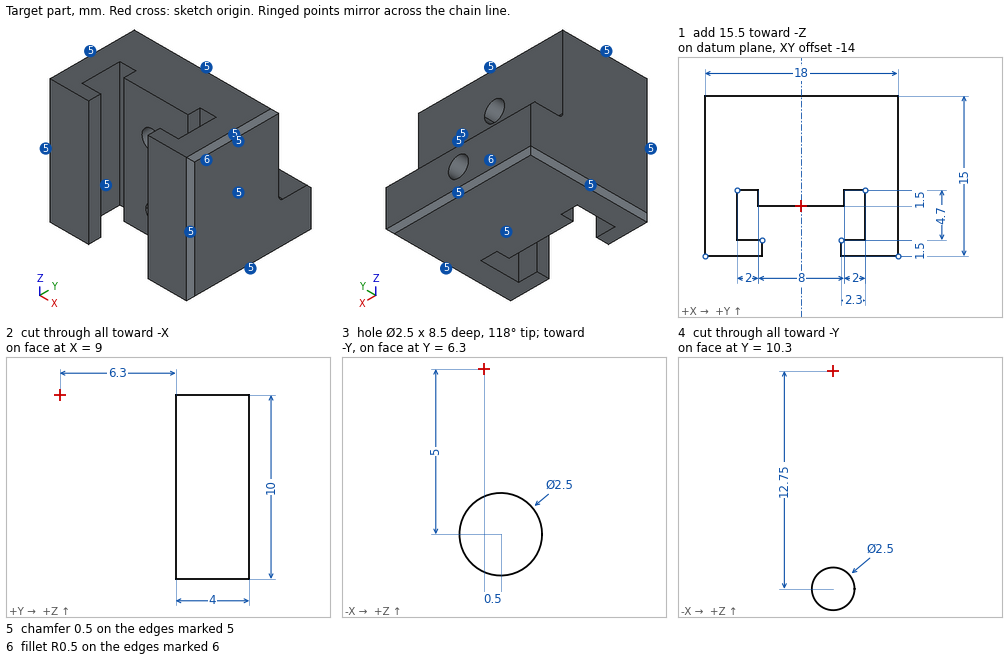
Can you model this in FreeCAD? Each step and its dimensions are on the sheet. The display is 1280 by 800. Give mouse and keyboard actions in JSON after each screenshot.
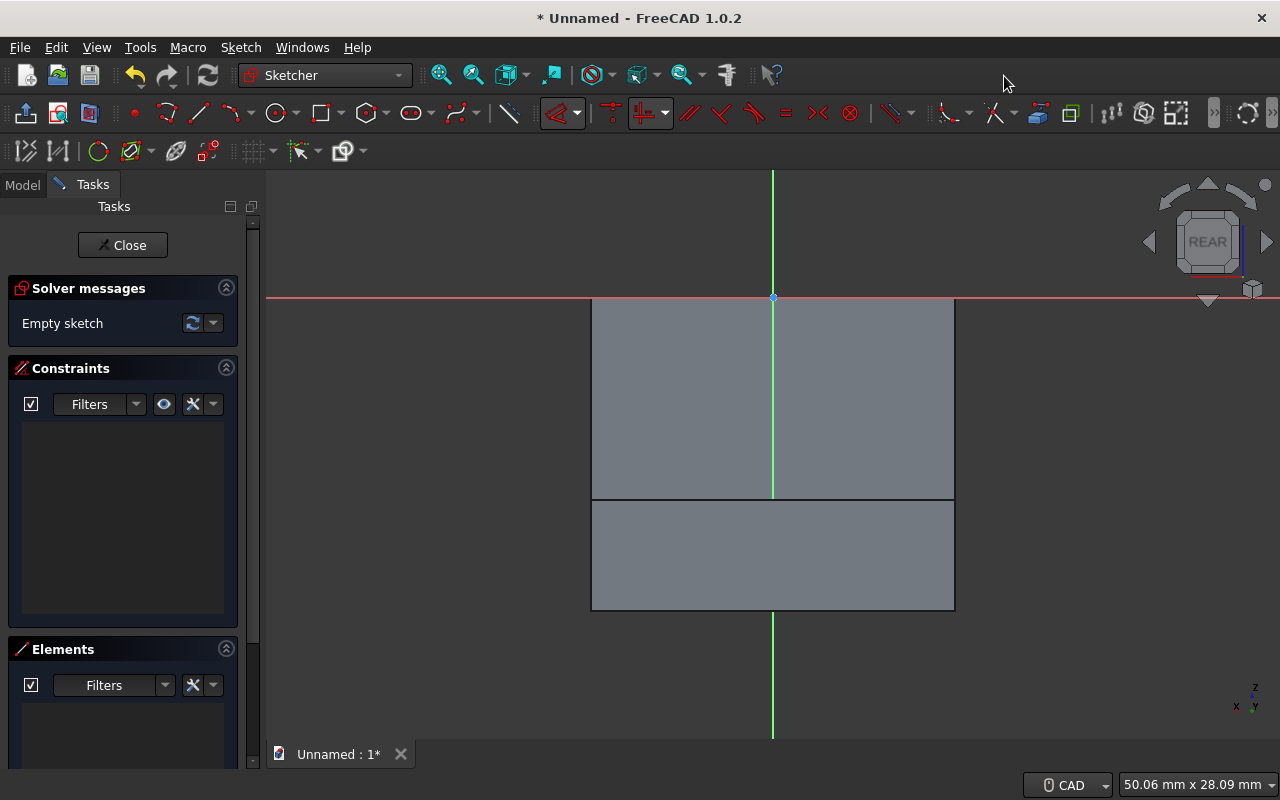
{"action": "scroll", "coordinate": [795, 390], "scroll_direction": "up", "scroll_amount": 10}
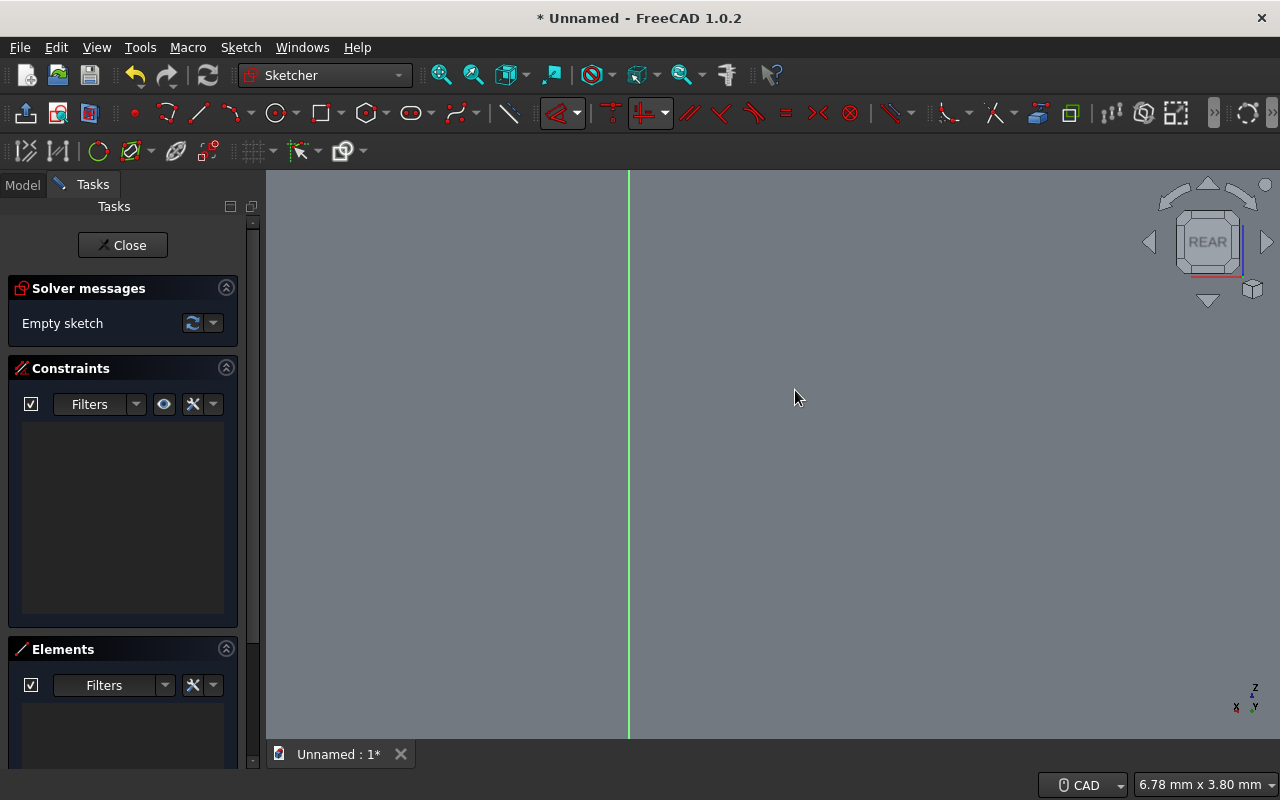
{"action": "key", "text": "g c"}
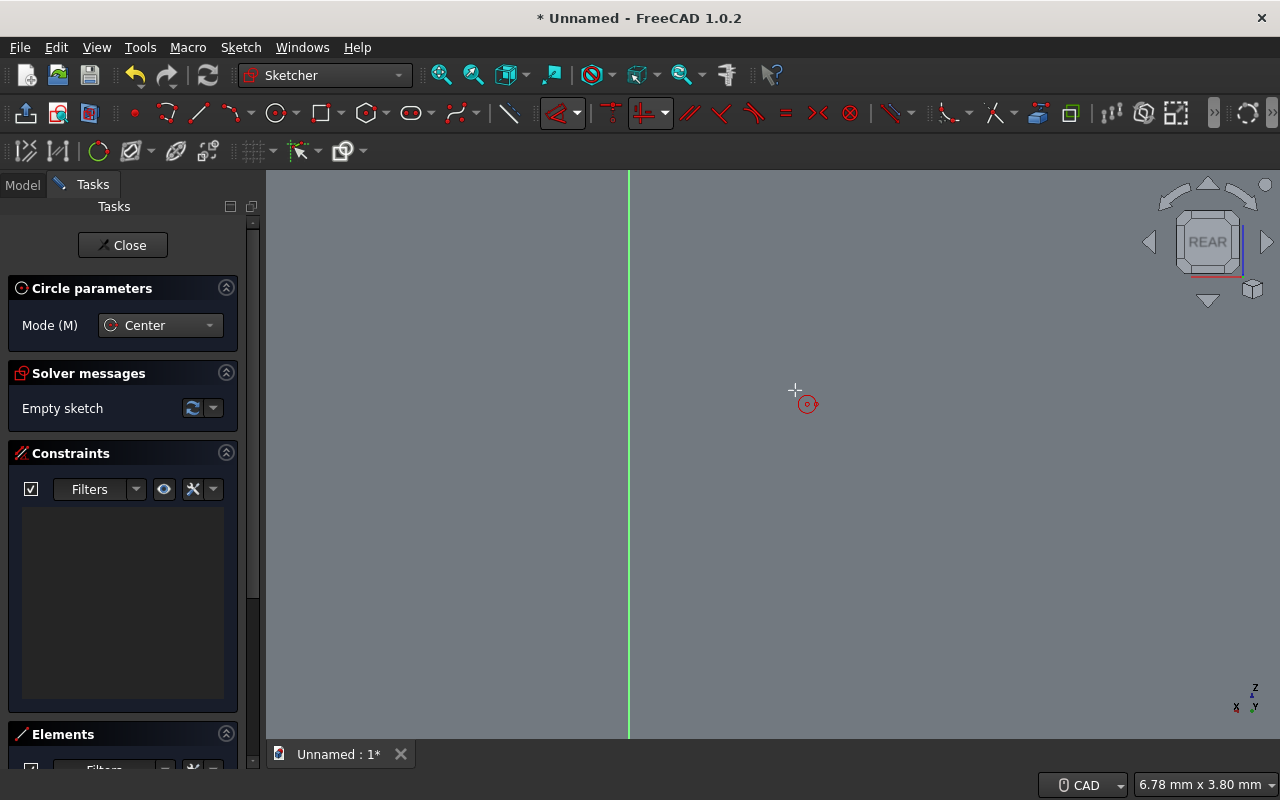
{"action": "left_click", "coordinate": [704, 453]}
{"action": "mouse_move", "coordinate": [836, 320]}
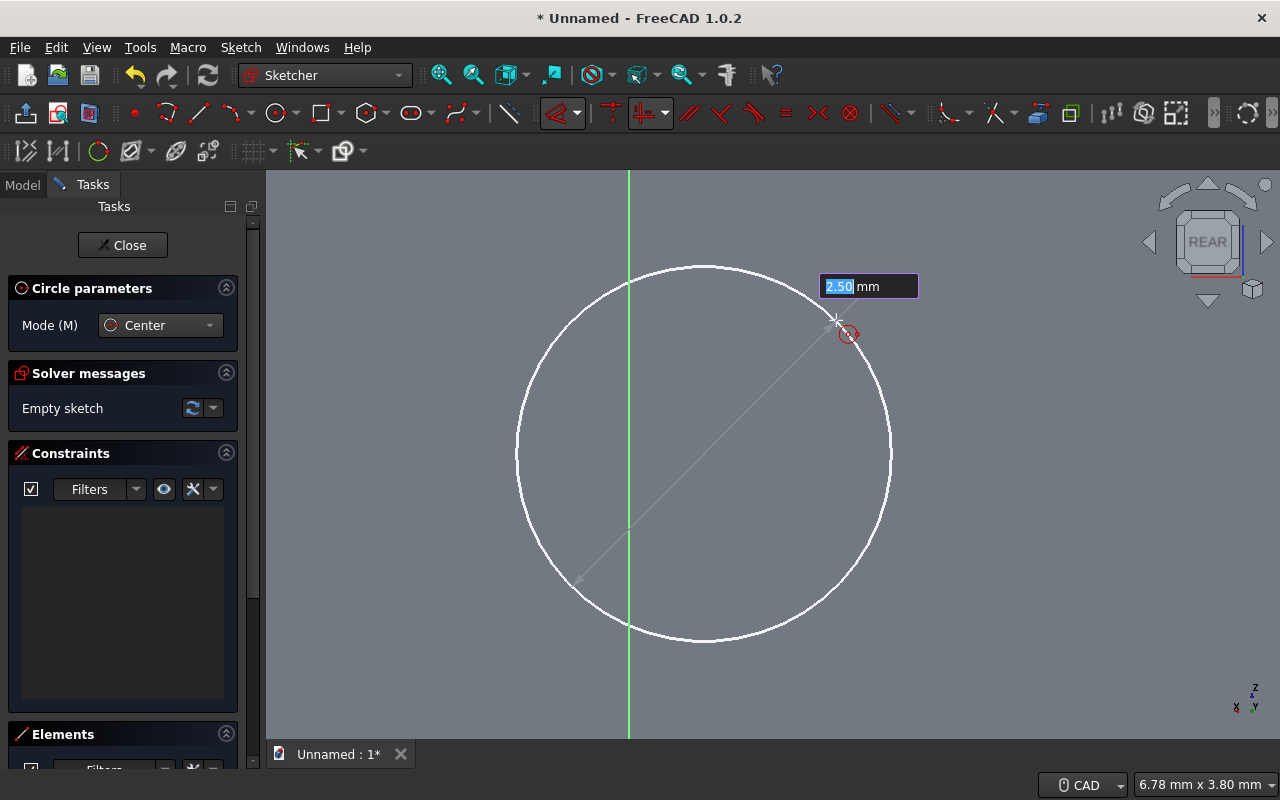
{"action": "type", "text": "2.5"}
{"action": "key", "text": "Return"}
{"action": "key", "text": "Escape"}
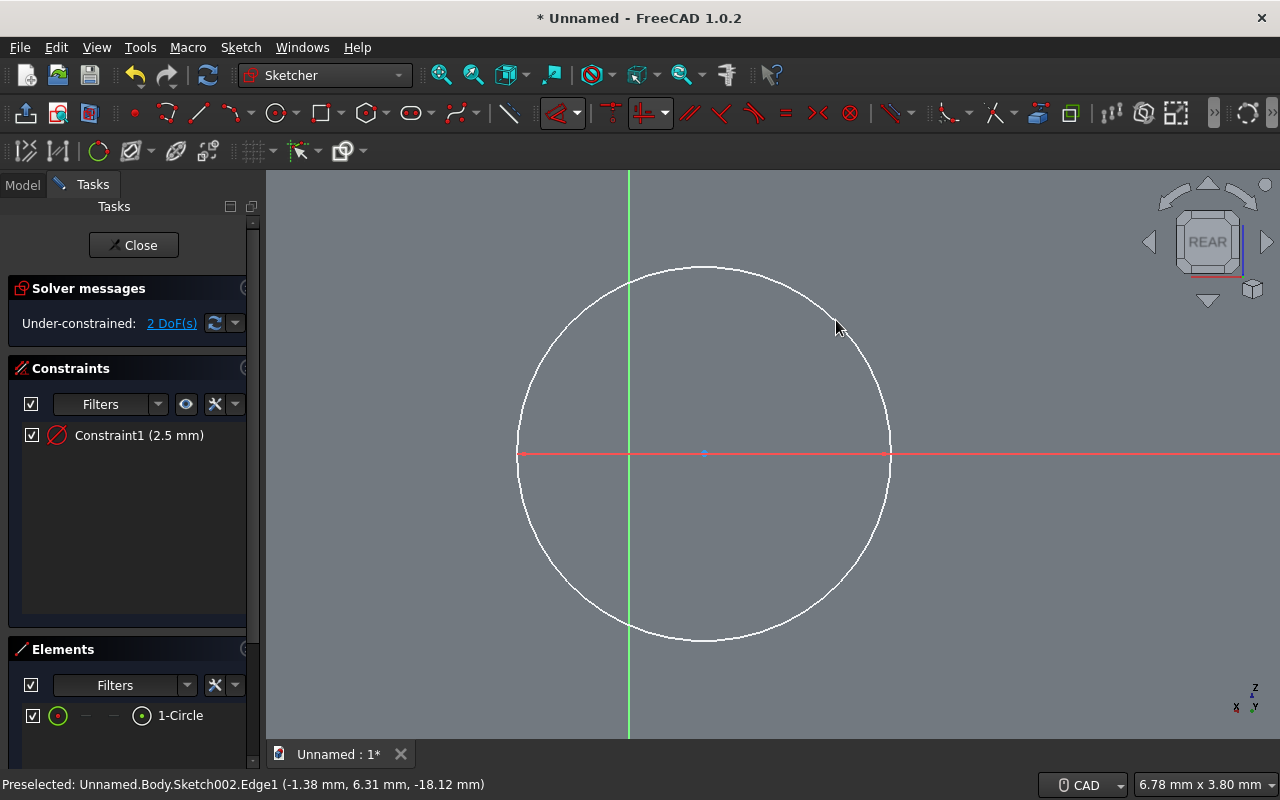
{"action": "left_click", "coordinate": [556, 114]}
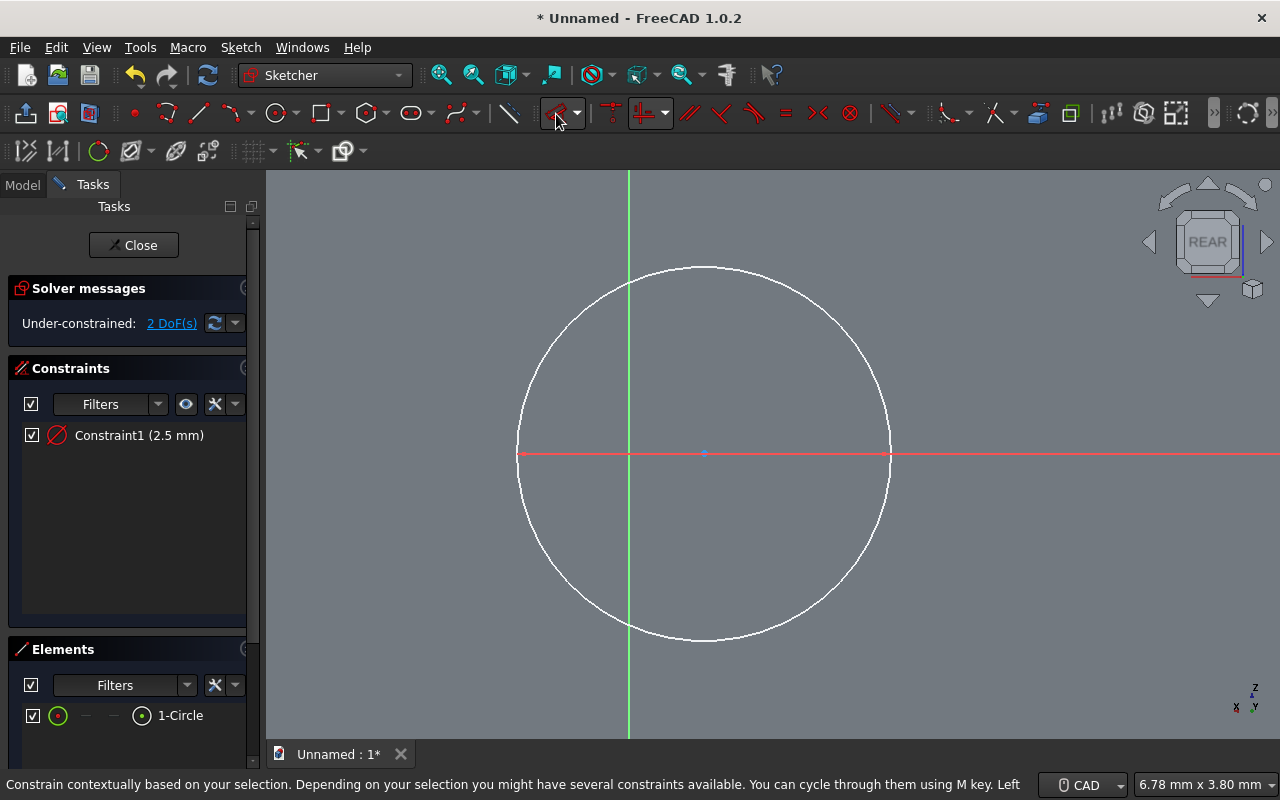
{"action": "left_click", "coordinate": [704, 454]}
{"action": "left_click", "coordinate": [595, 326]}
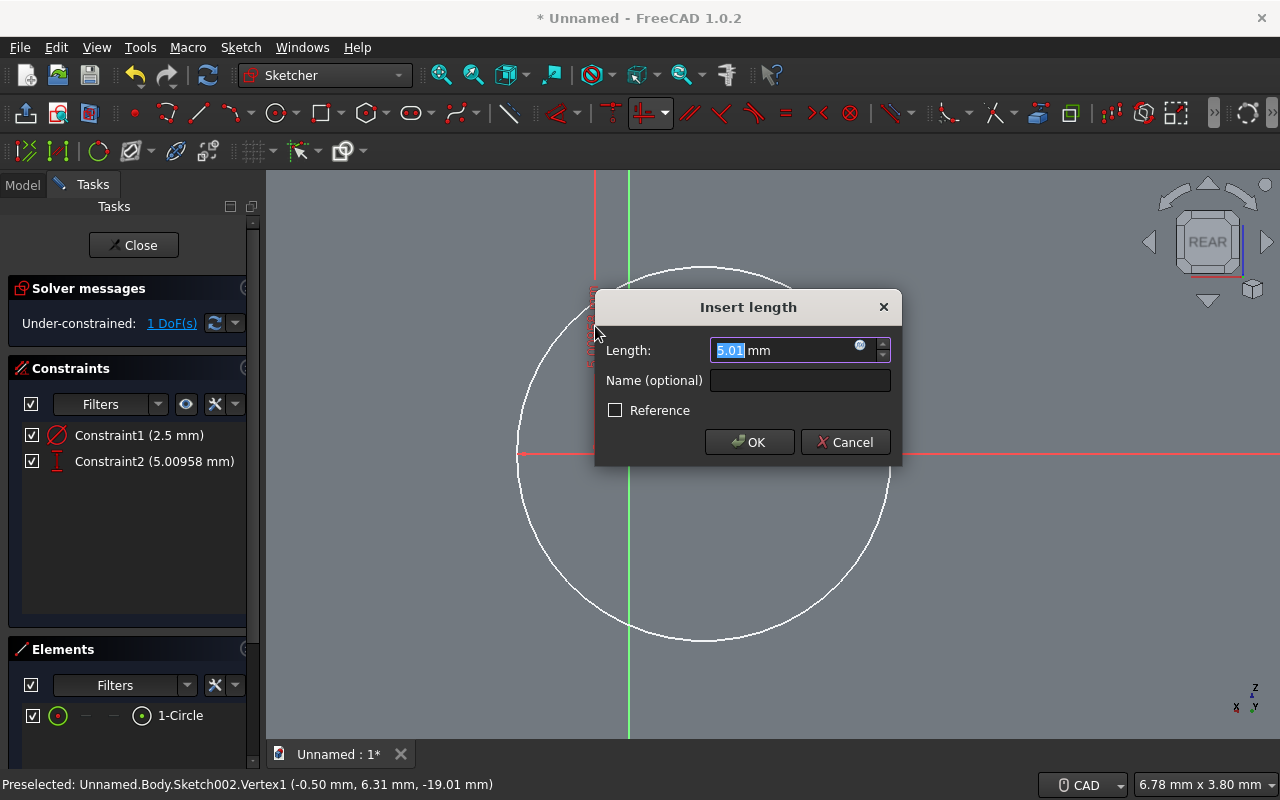
{"action": "type", "text": "5"}
{"action": "key", "text": "Return"}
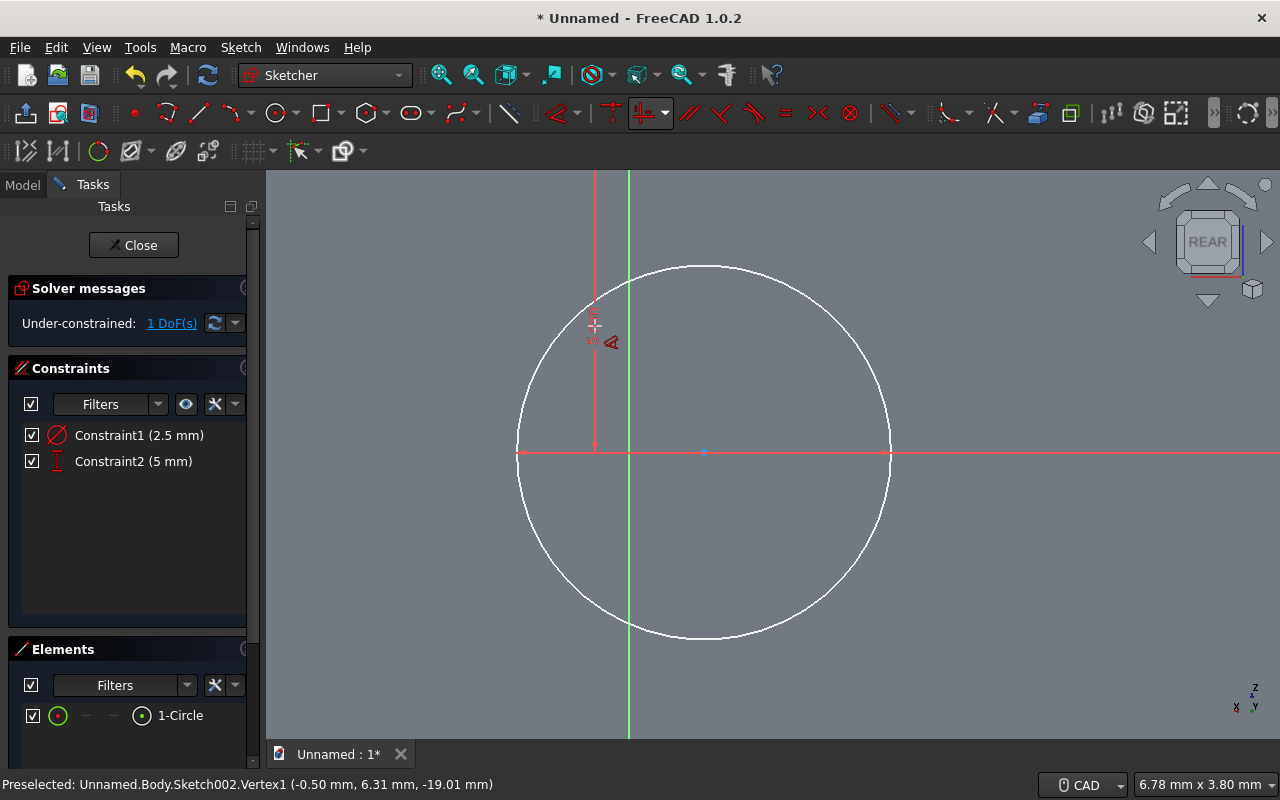
{"action": "left_click", "coordinate": [704, 453]}
{"action": "left_click", "coordinate": [667, 487]}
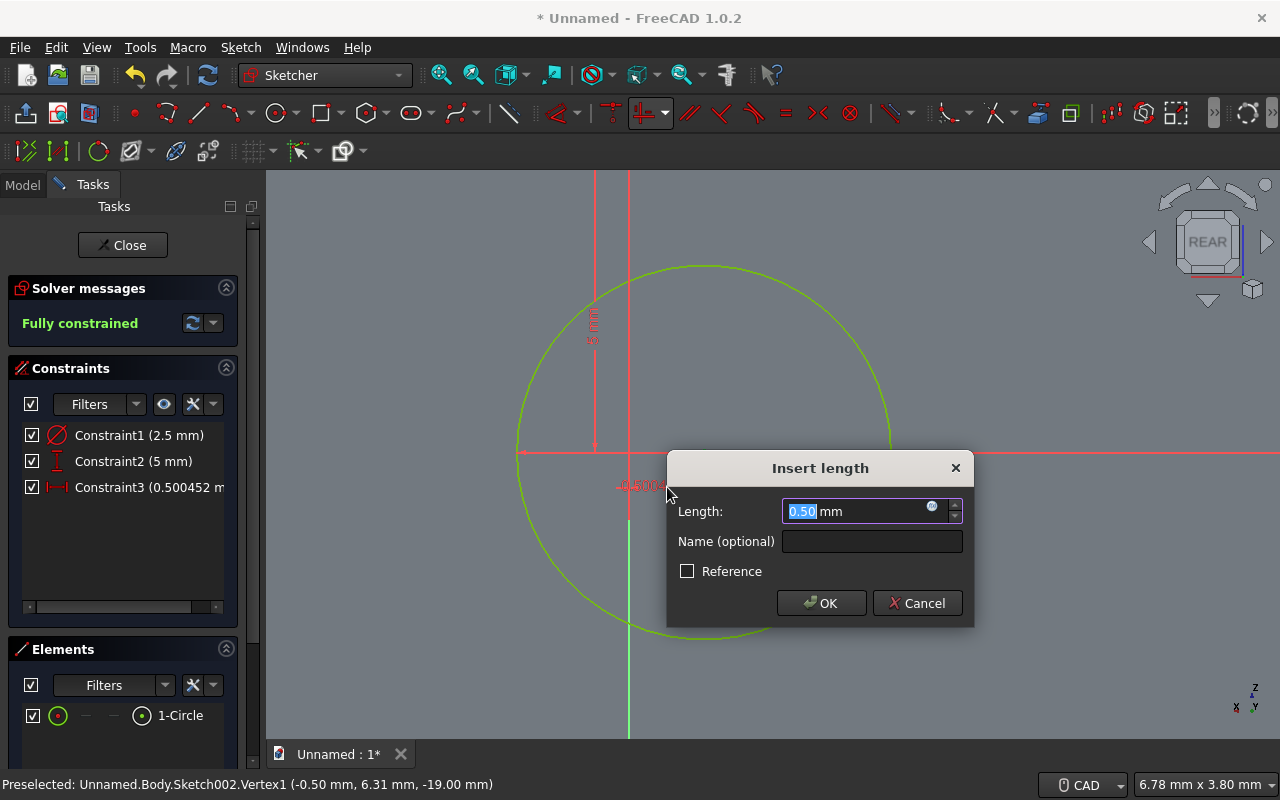
{"action": "type", "text": "0.5"}
{"action": "key", "text": "Return"}
{"action": "key", "text": "Escape"}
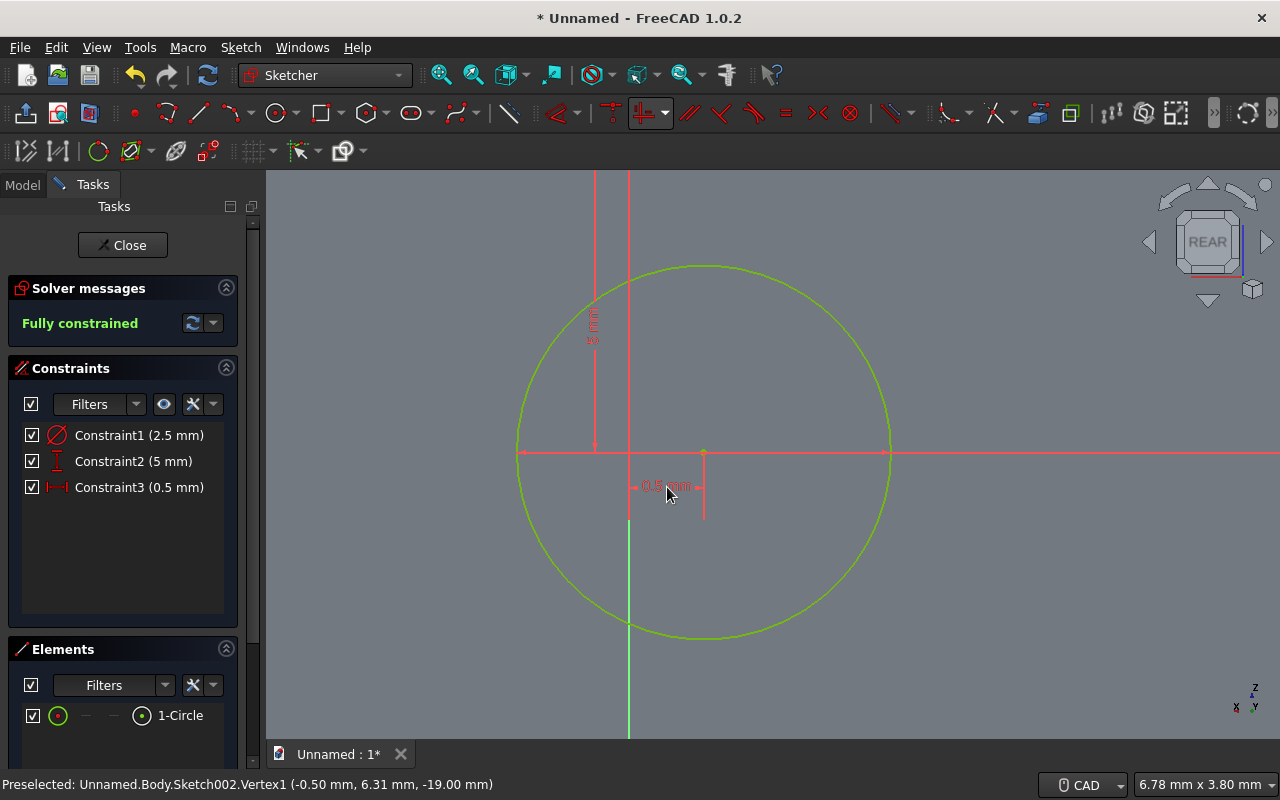
{"action": "left_click", "coordinate": [123, 245]}